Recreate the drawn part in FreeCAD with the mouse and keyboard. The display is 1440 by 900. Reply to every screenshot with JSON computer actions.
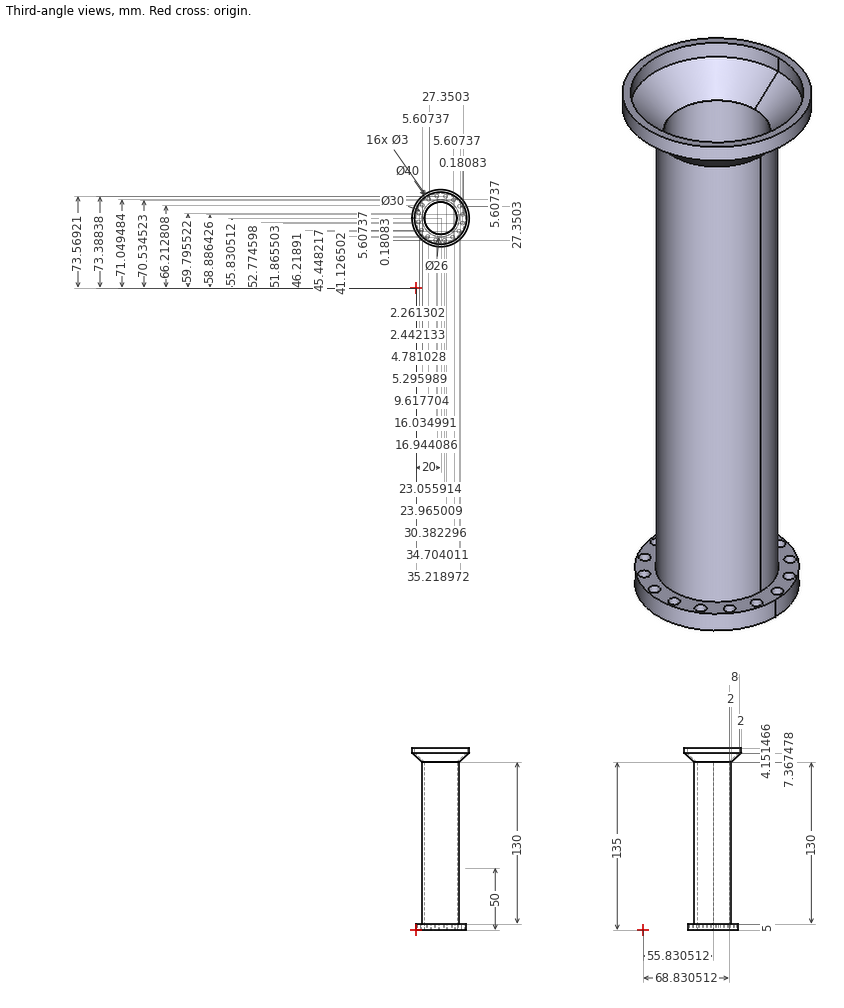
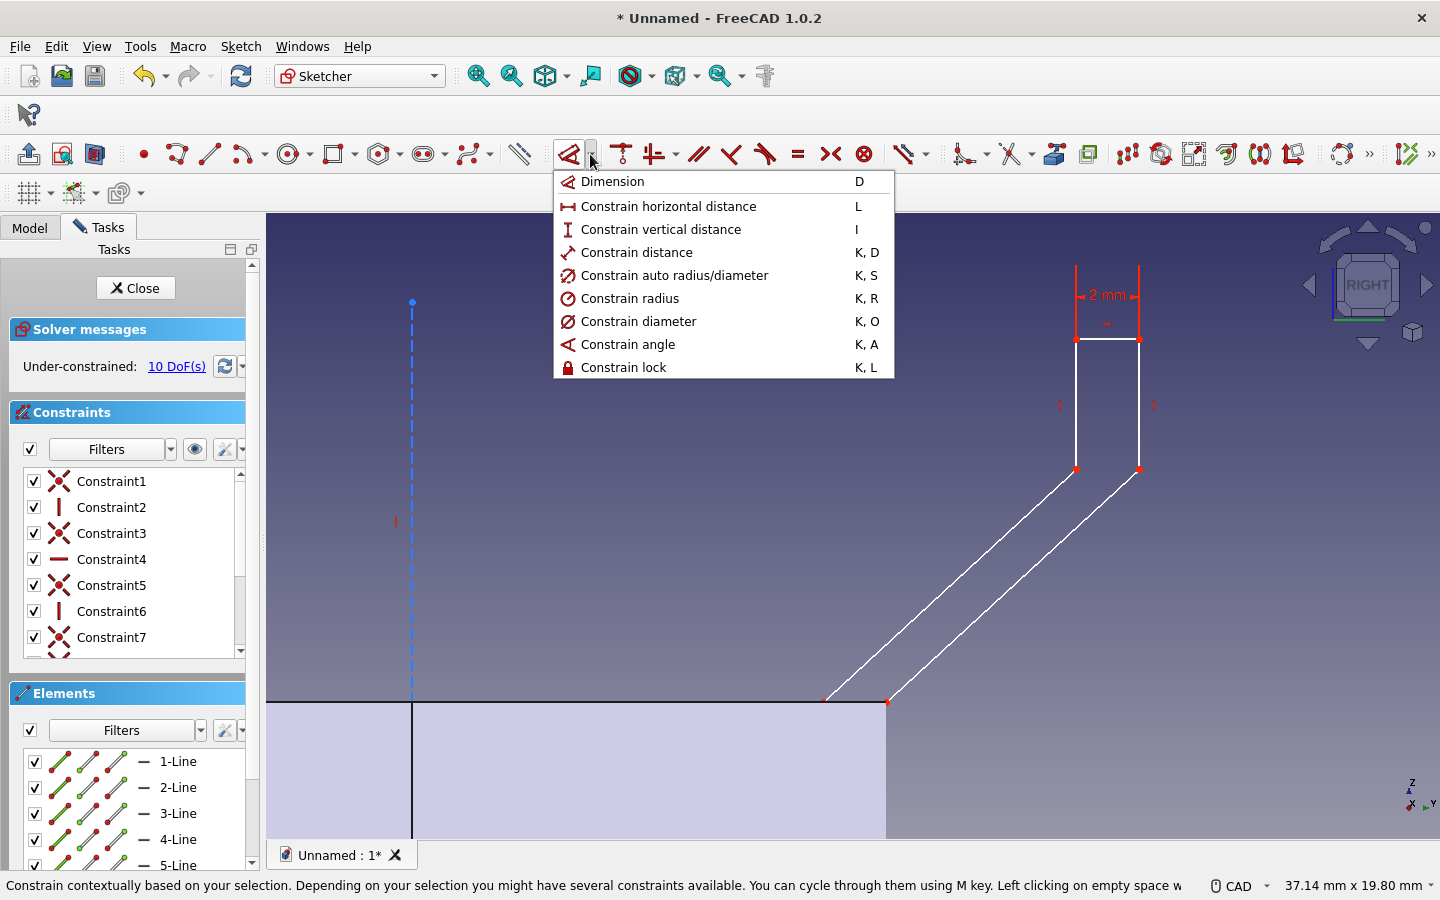
{"action": "left_click", "coordinate": [724, 206]}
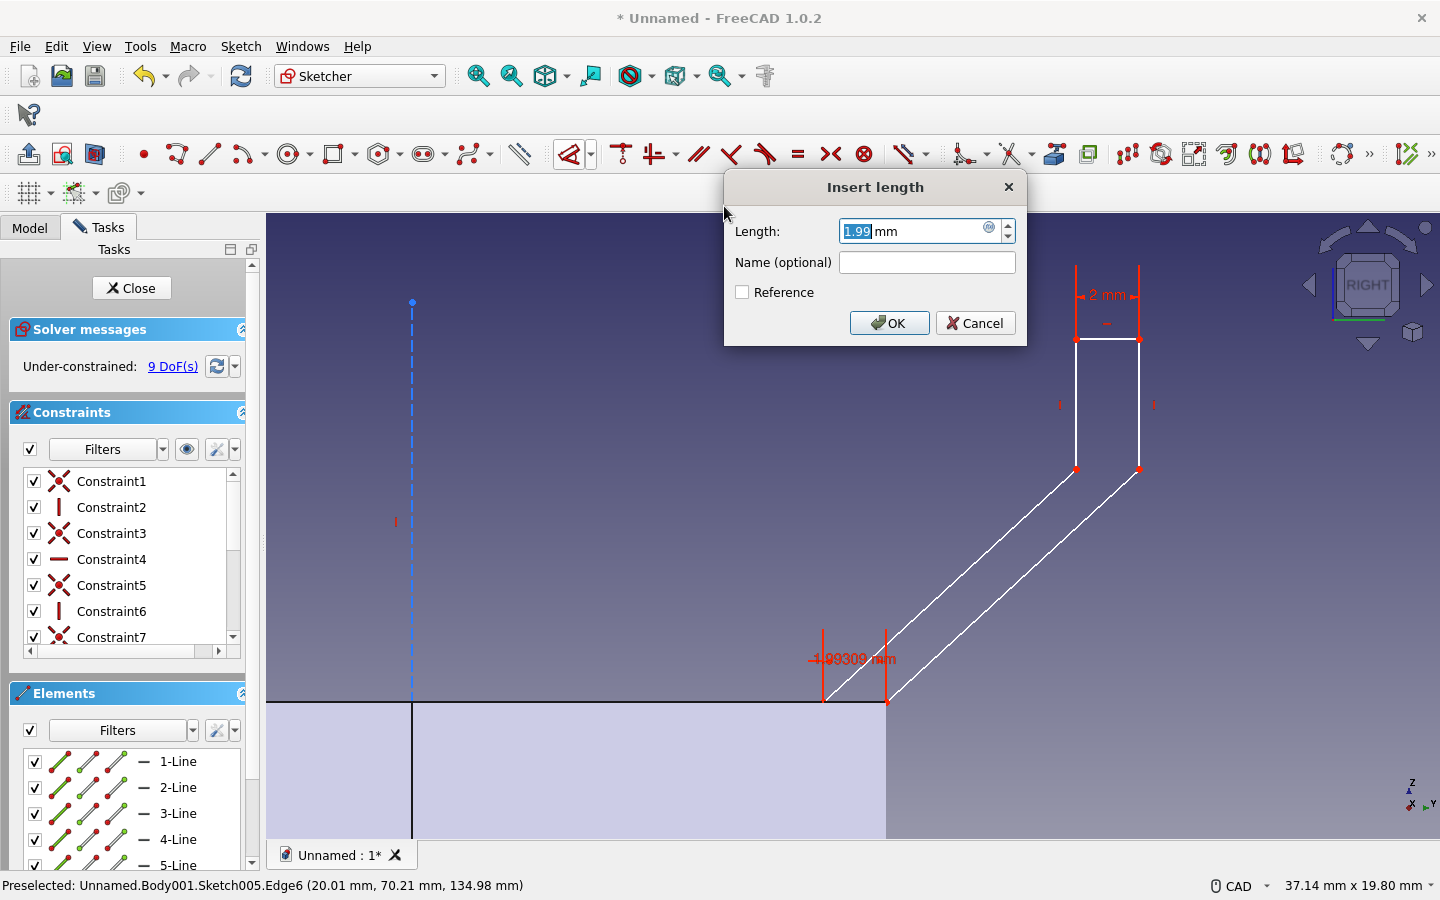
{"action": "type", "text": "2"}
{"action": "key", "text": "Return"}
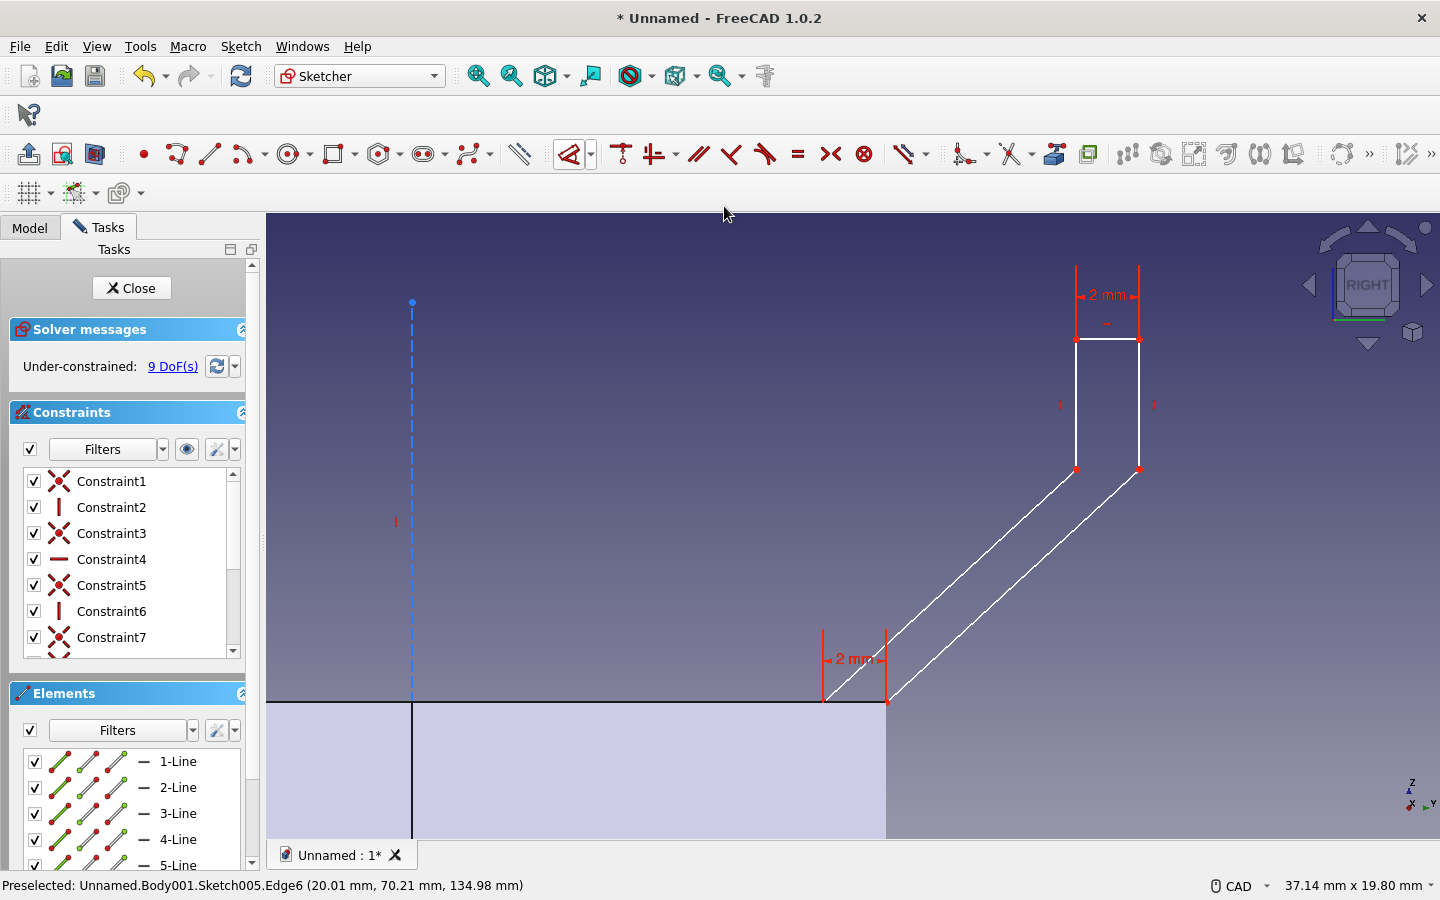
{"action": "left_click", "coordinate": [899, 633]}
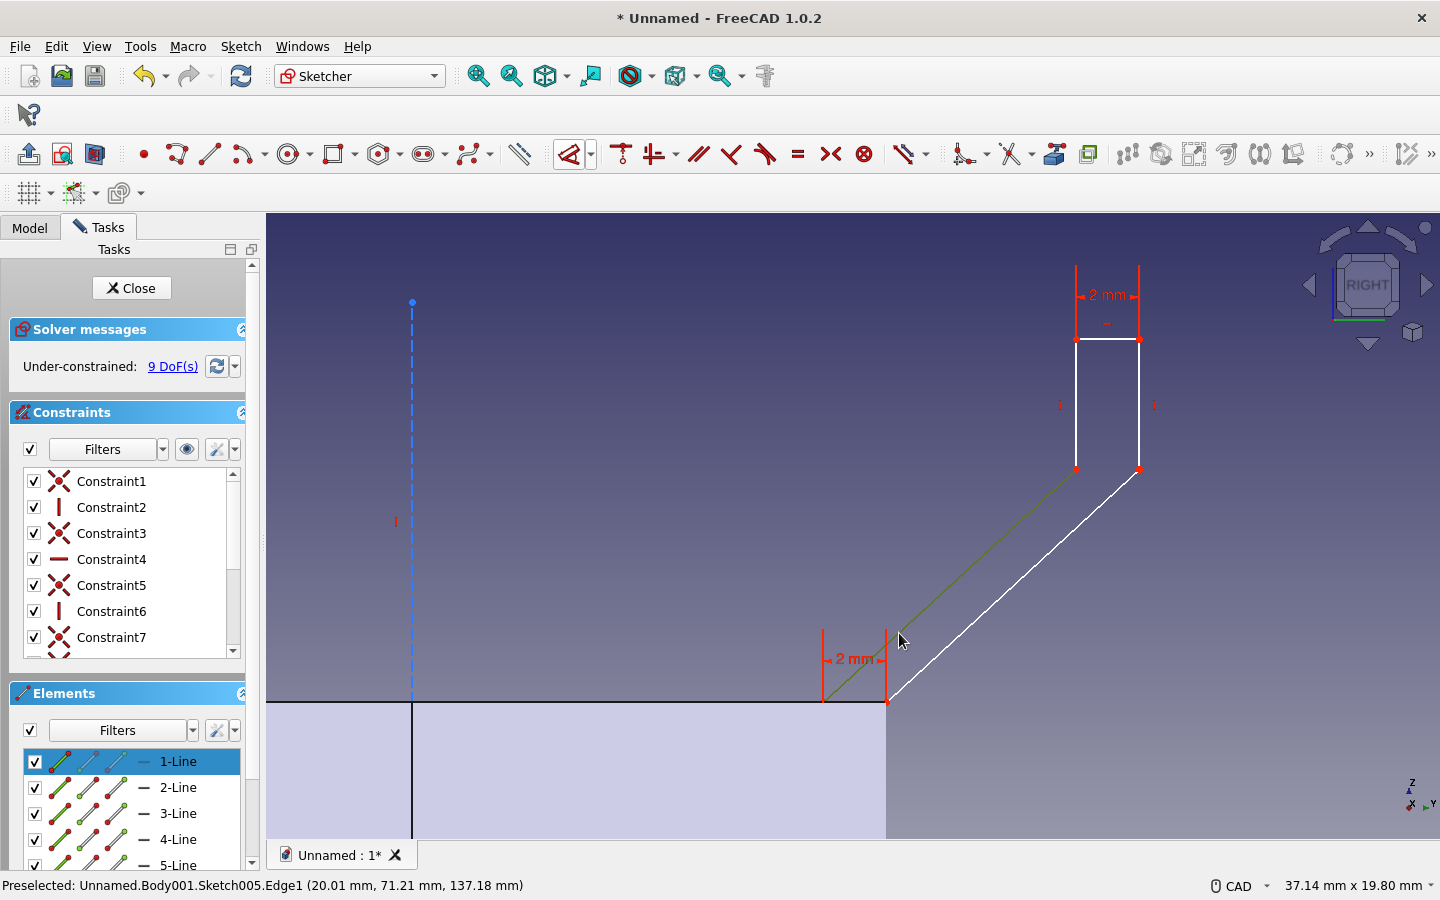
{"action": "key", "text": "l"}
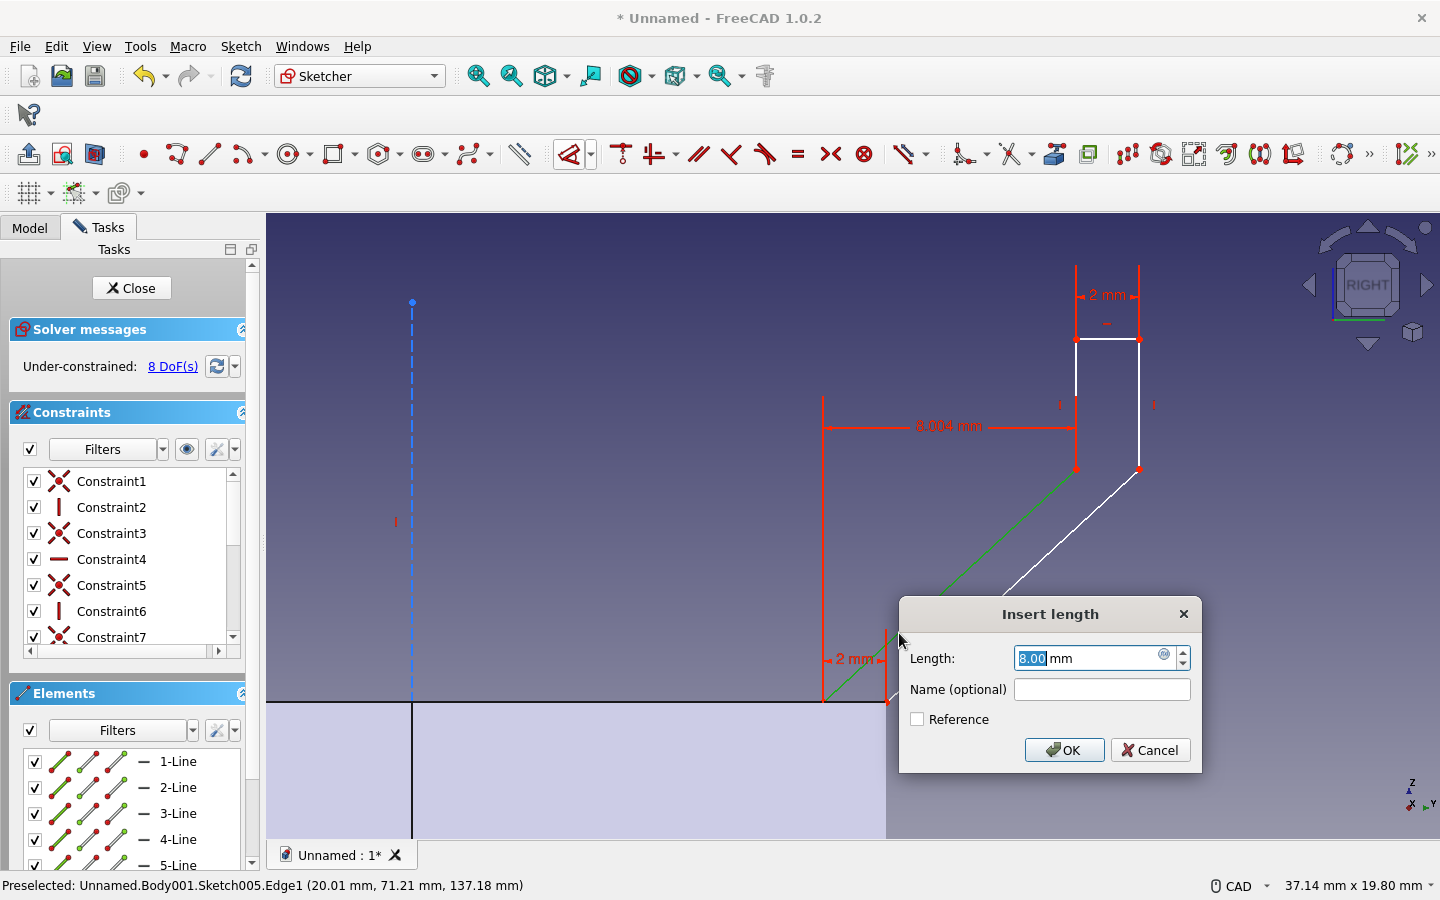
{"action": "type", "text": "8"}
{"action": "key", "text": "Return"}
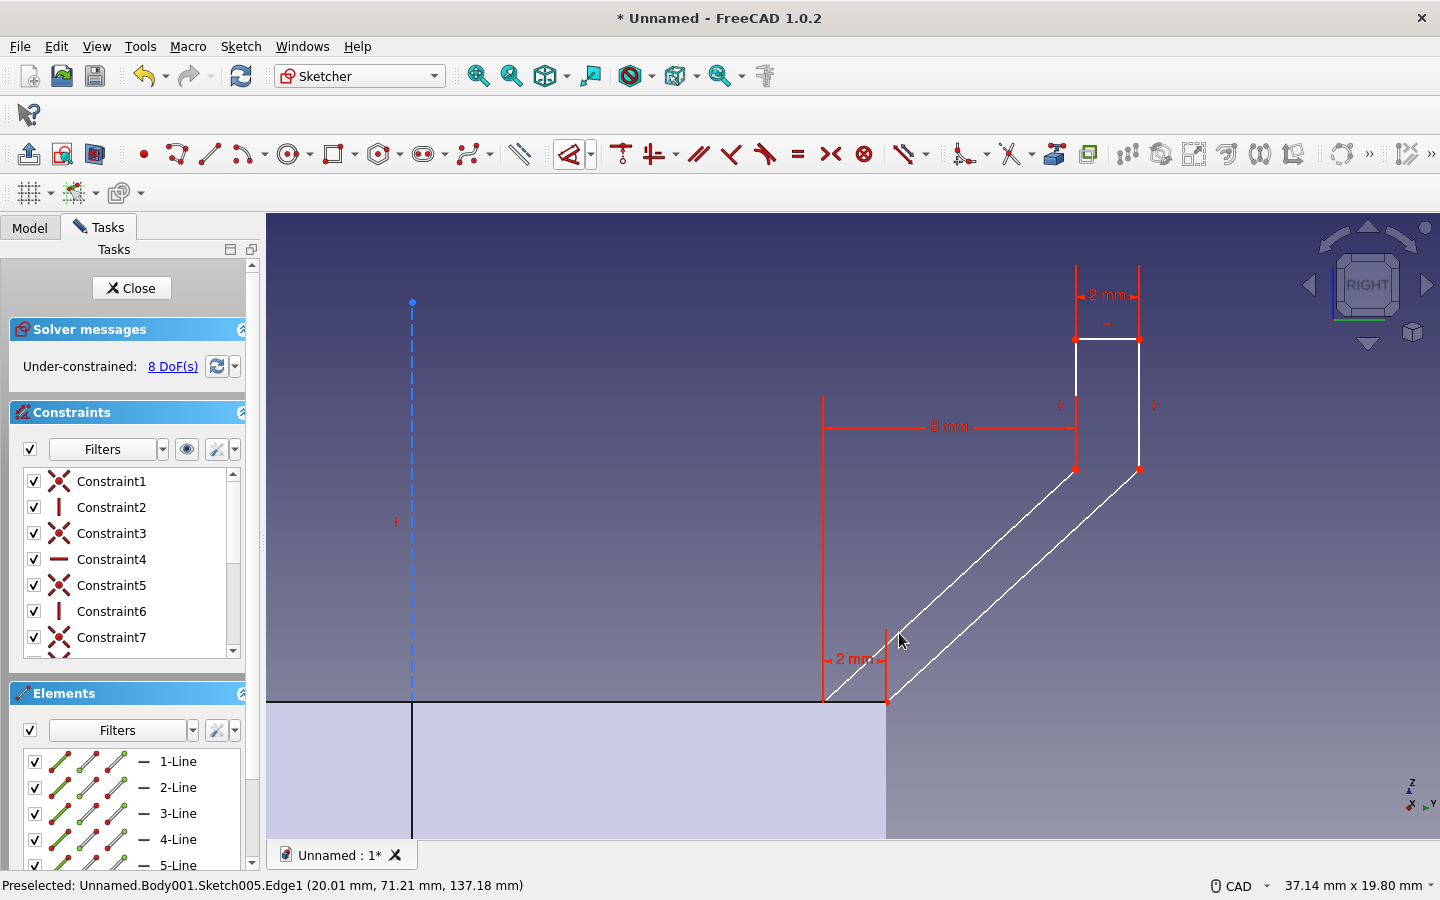
{"action": "left_click", "coordinate": [823, 703]}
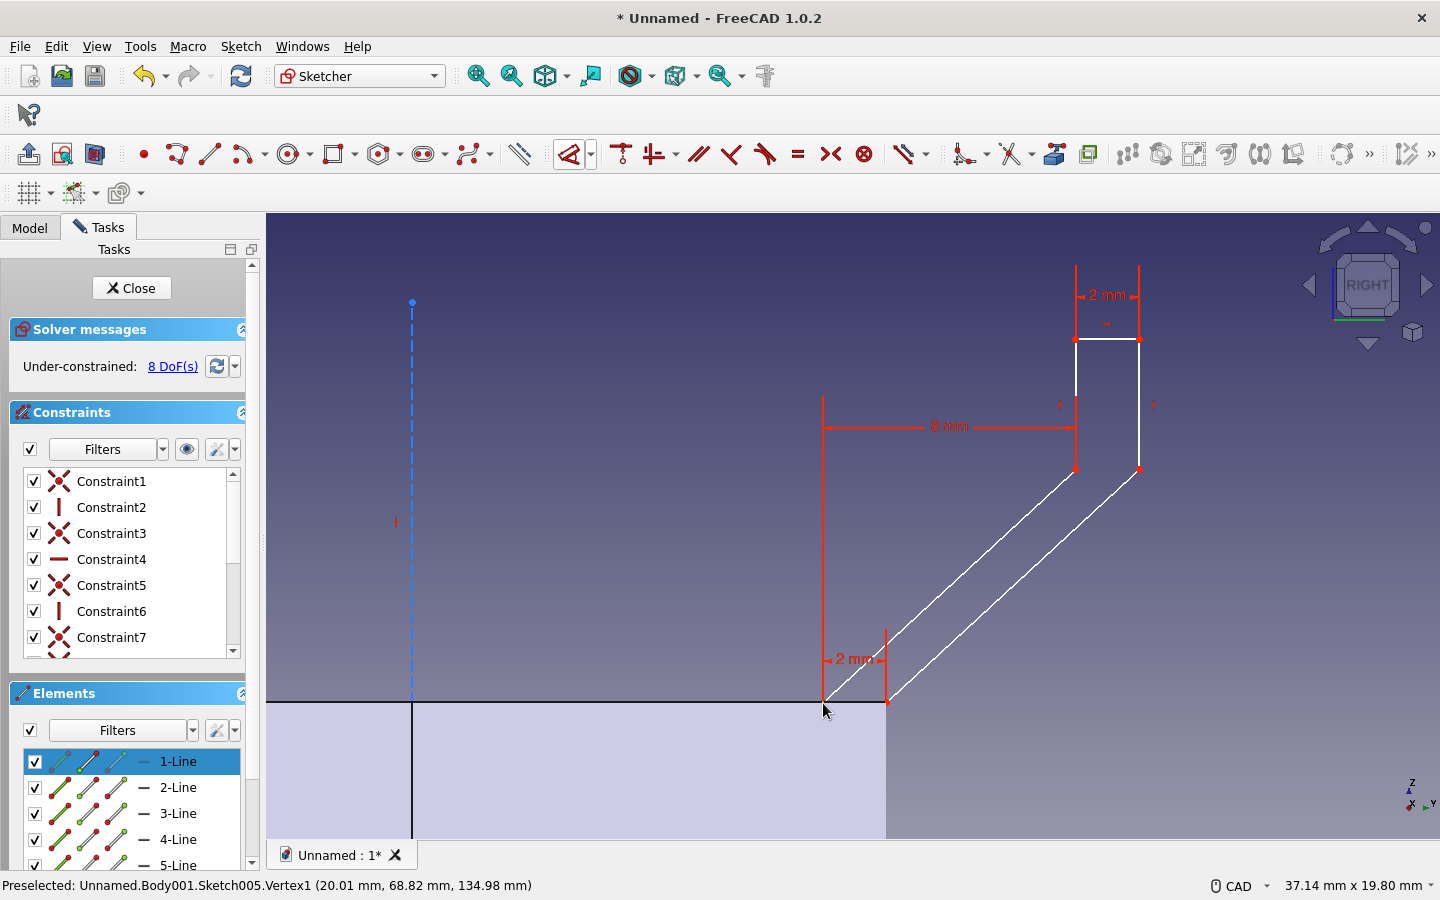
{"action": "left_click", "coordinate": [590, 154]}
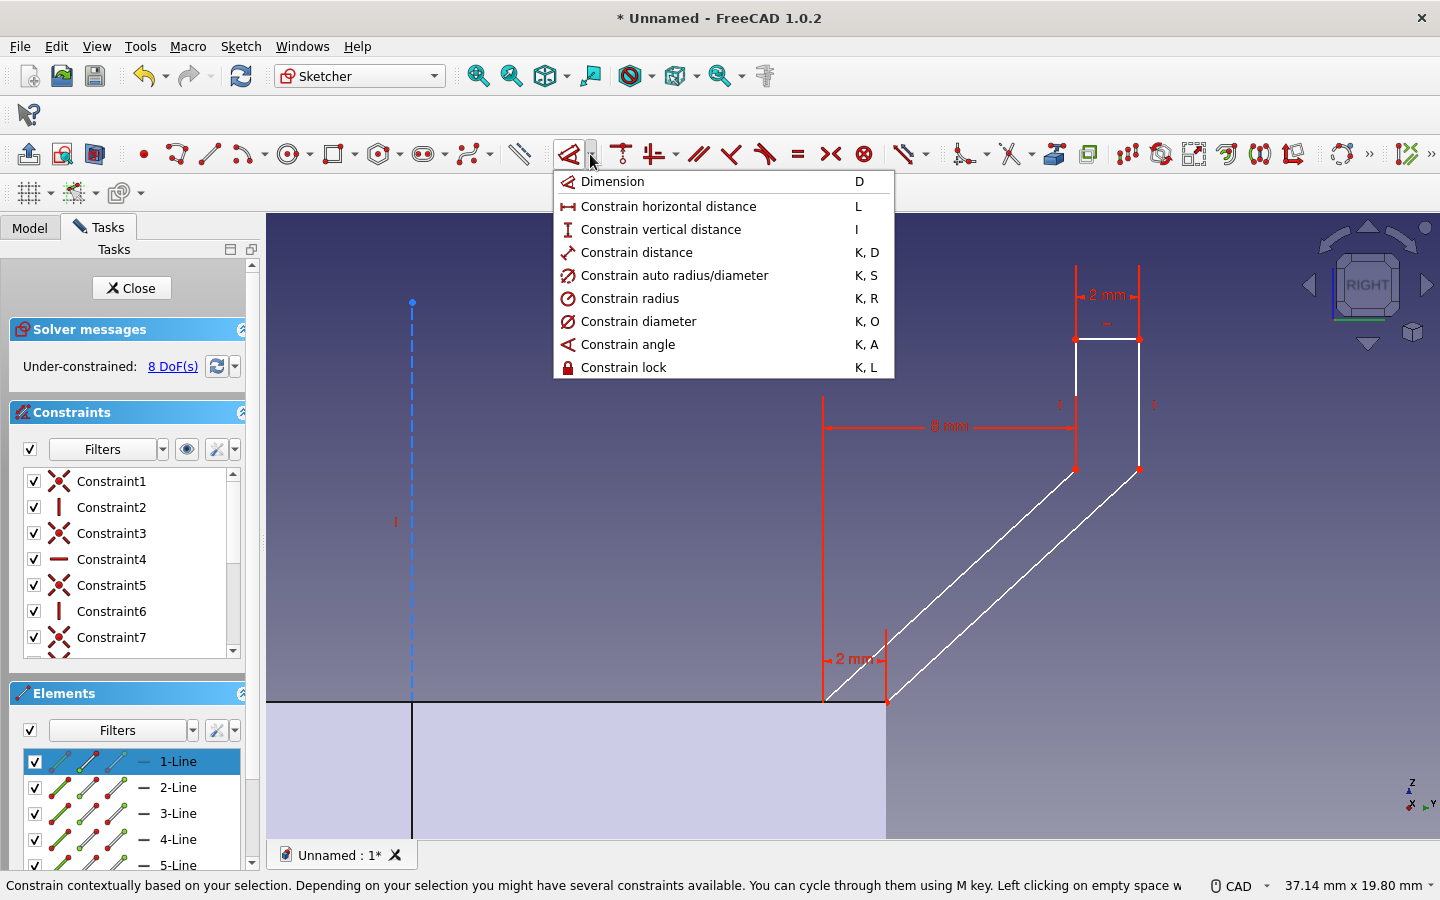
{"action": "left_click", "coordinate": [724, 230]}